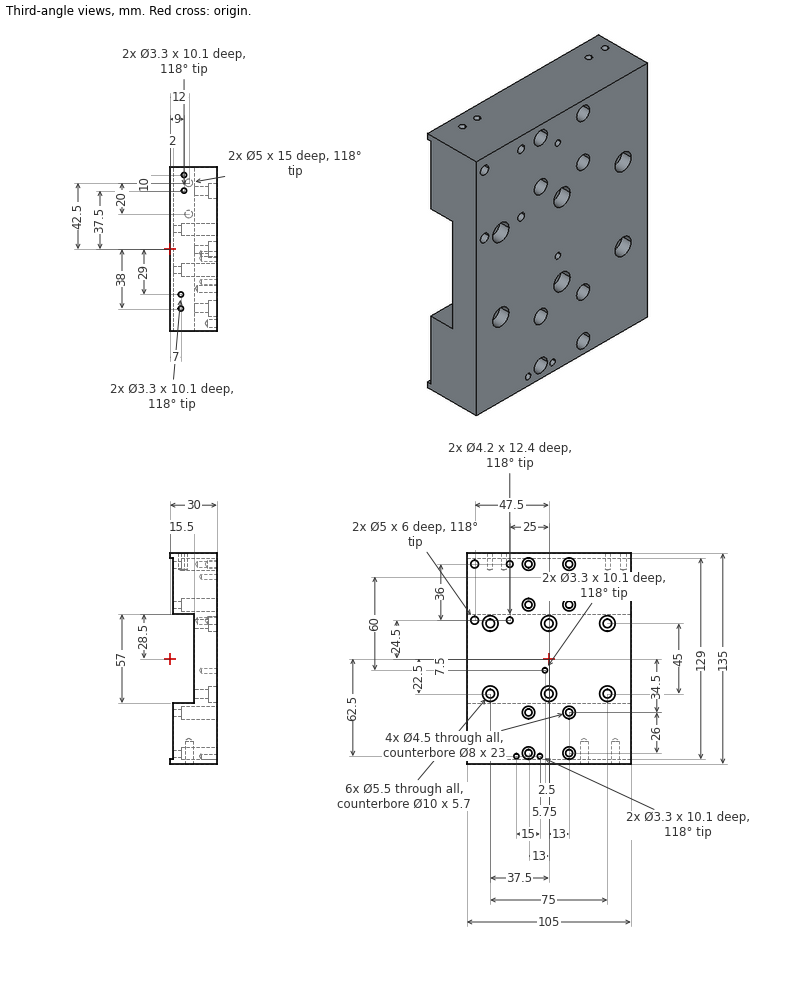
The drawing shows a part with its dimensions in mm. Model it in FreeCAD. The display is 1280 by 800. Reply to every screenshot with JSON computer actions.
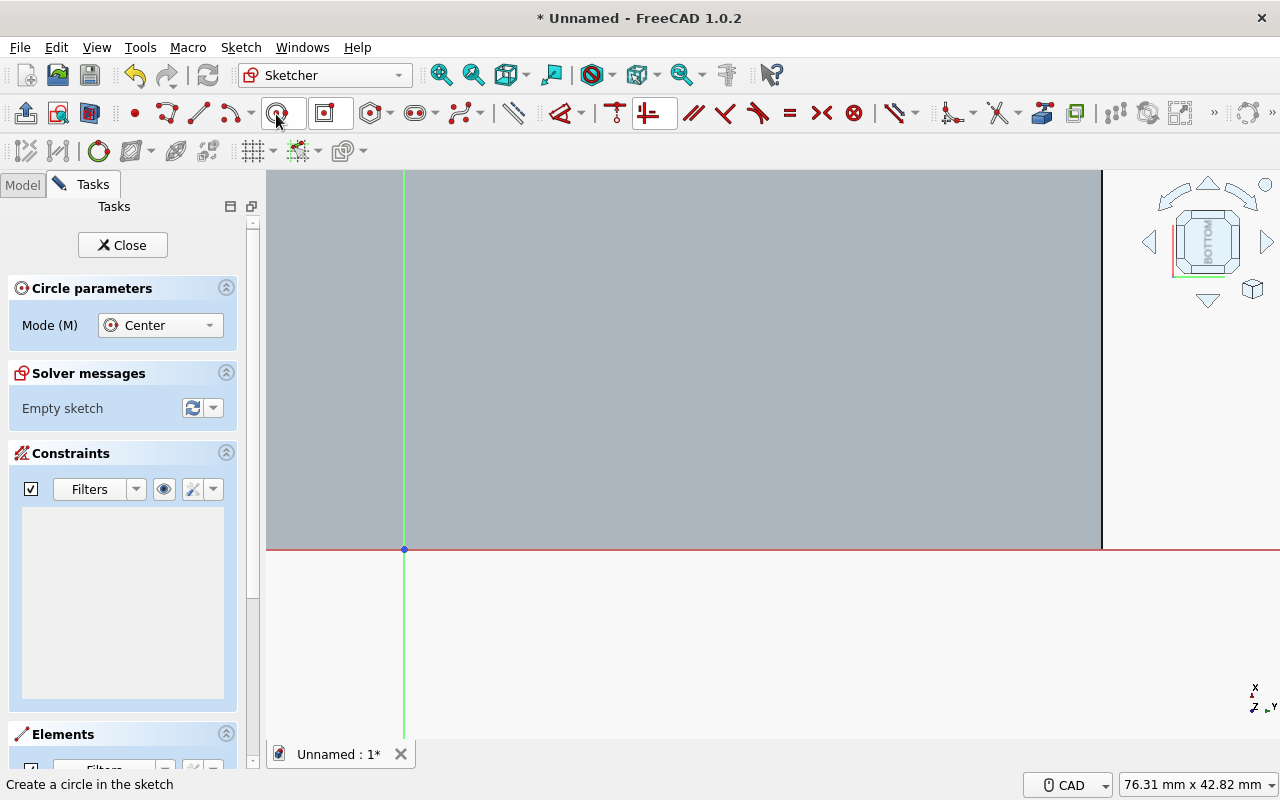
{"action": "left_click", "coordinate": [969, 390]}
{"action": "left_click", "coordinate": [993, 367]}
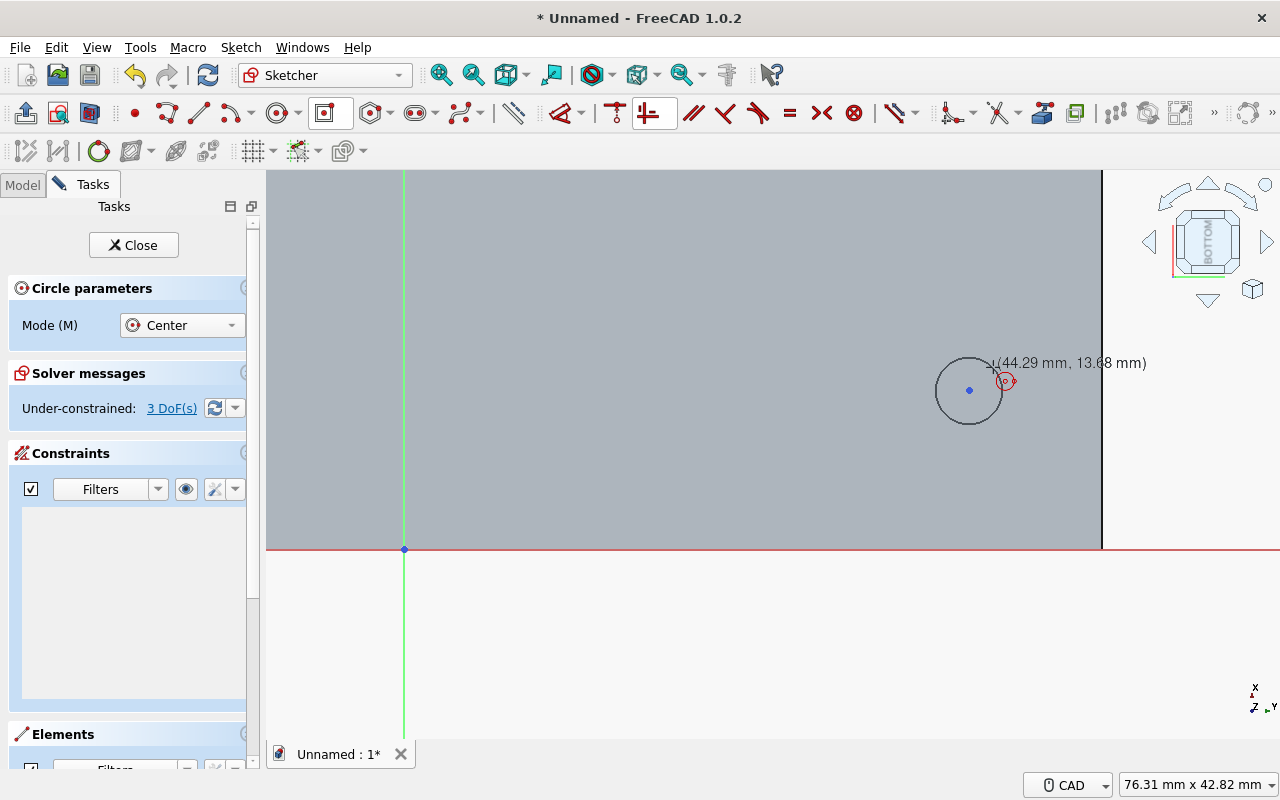
{"action": "left_click", "coordinate": [703, 390]}
{"action": "left_click", "coordinate": [727, 367]}
{"action": "key", "text": "Escape"}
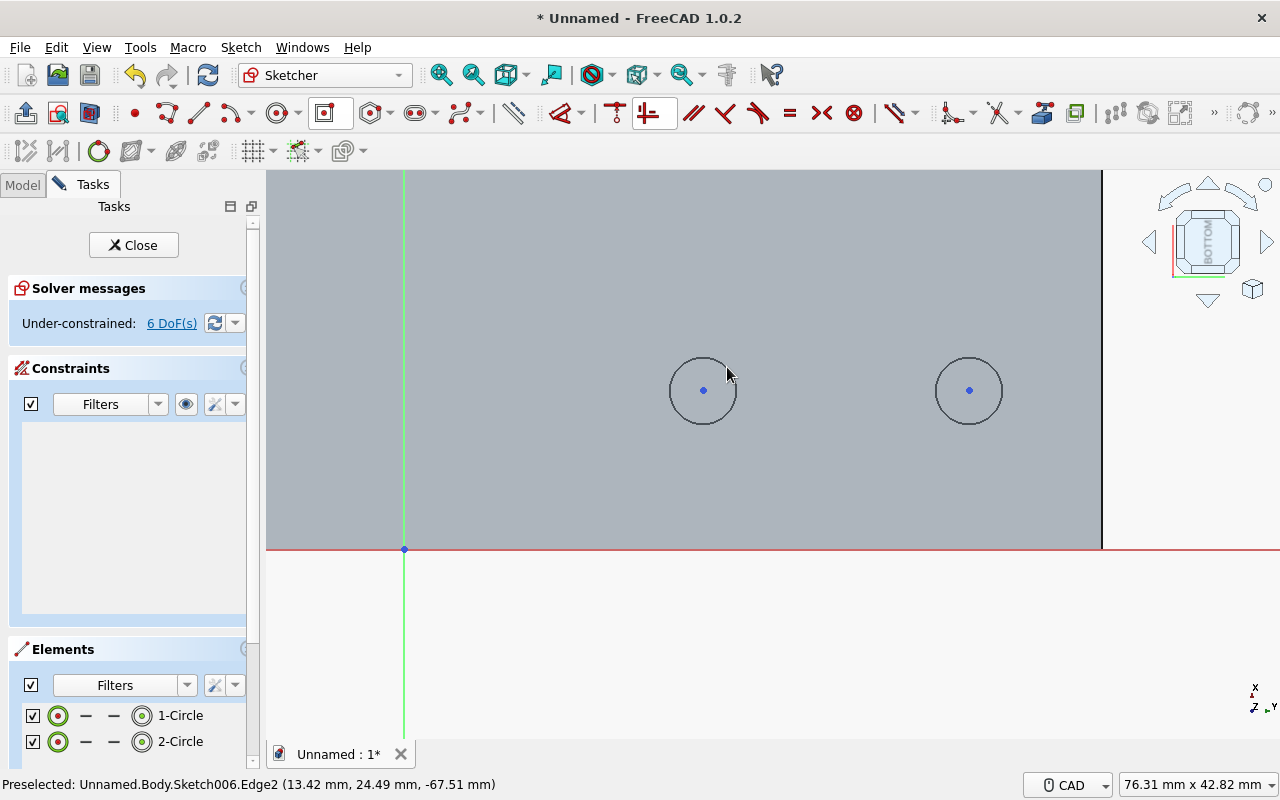
{"action": "left_click", "coordinate": [992, 367]}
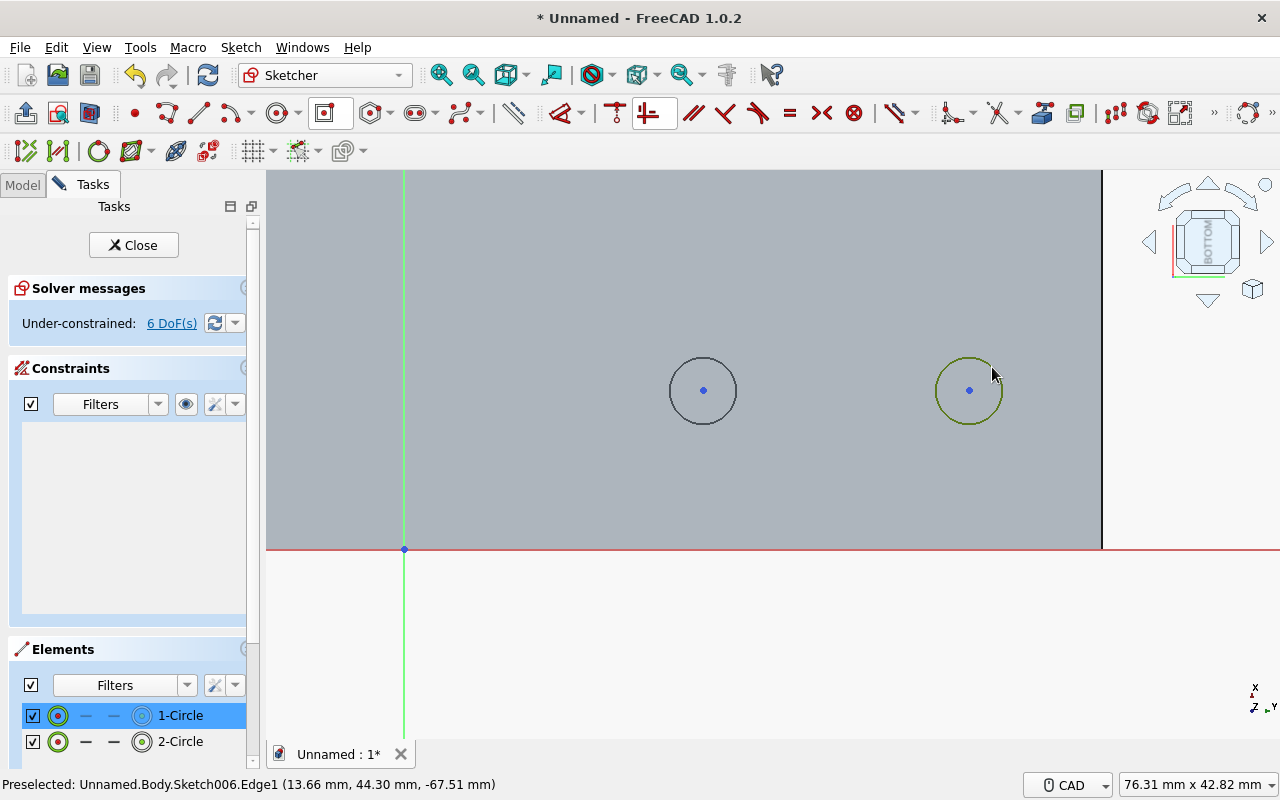
{"action": "left_click", "coordinate": [726, 367]}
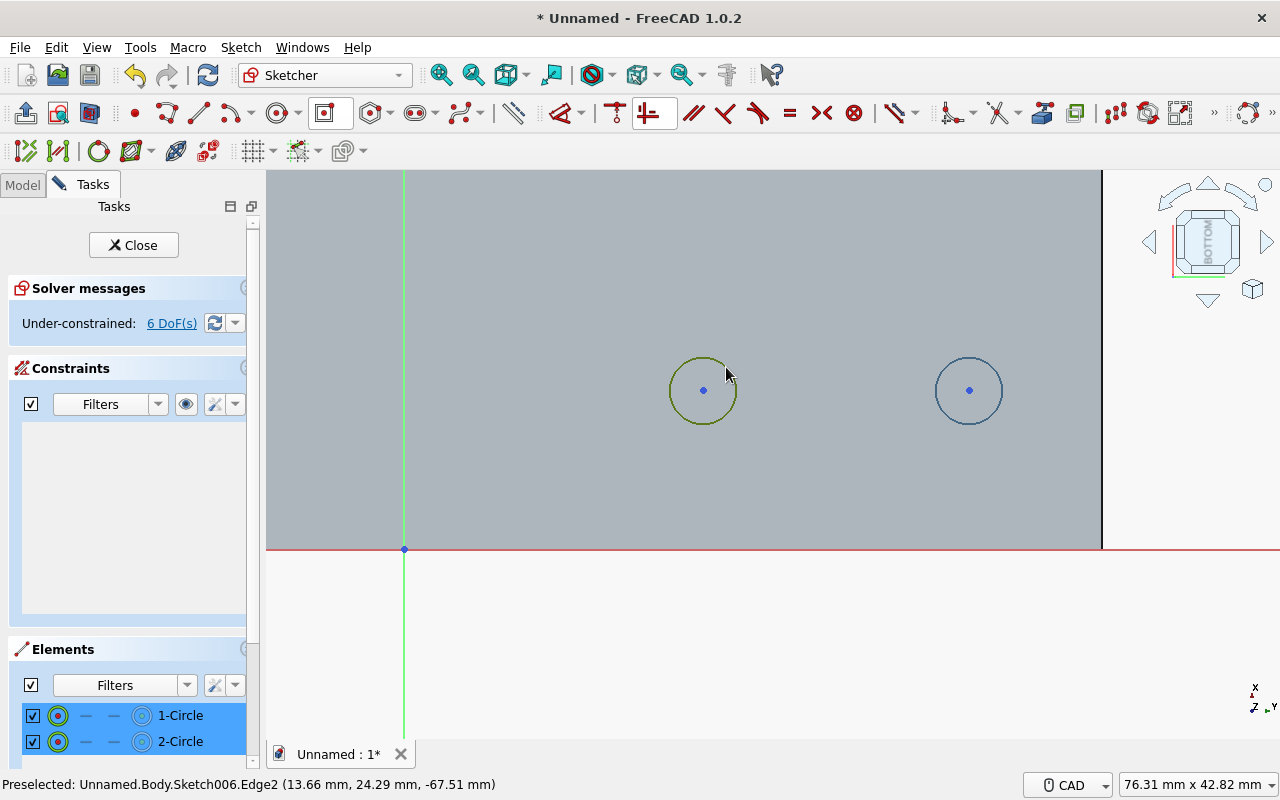
{"action": "left_click", "coordinate": [790, 114]}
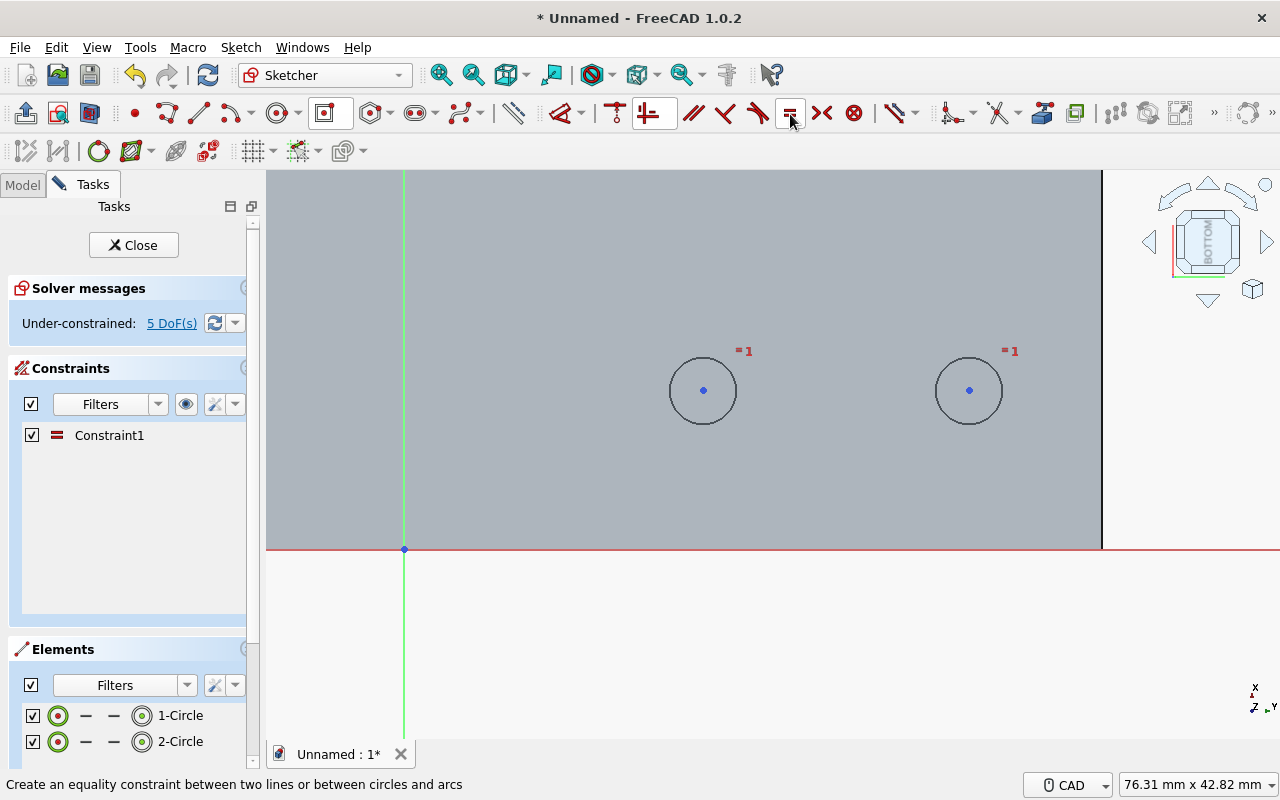
{"action": "left_click", "coordinate": [969, 391]}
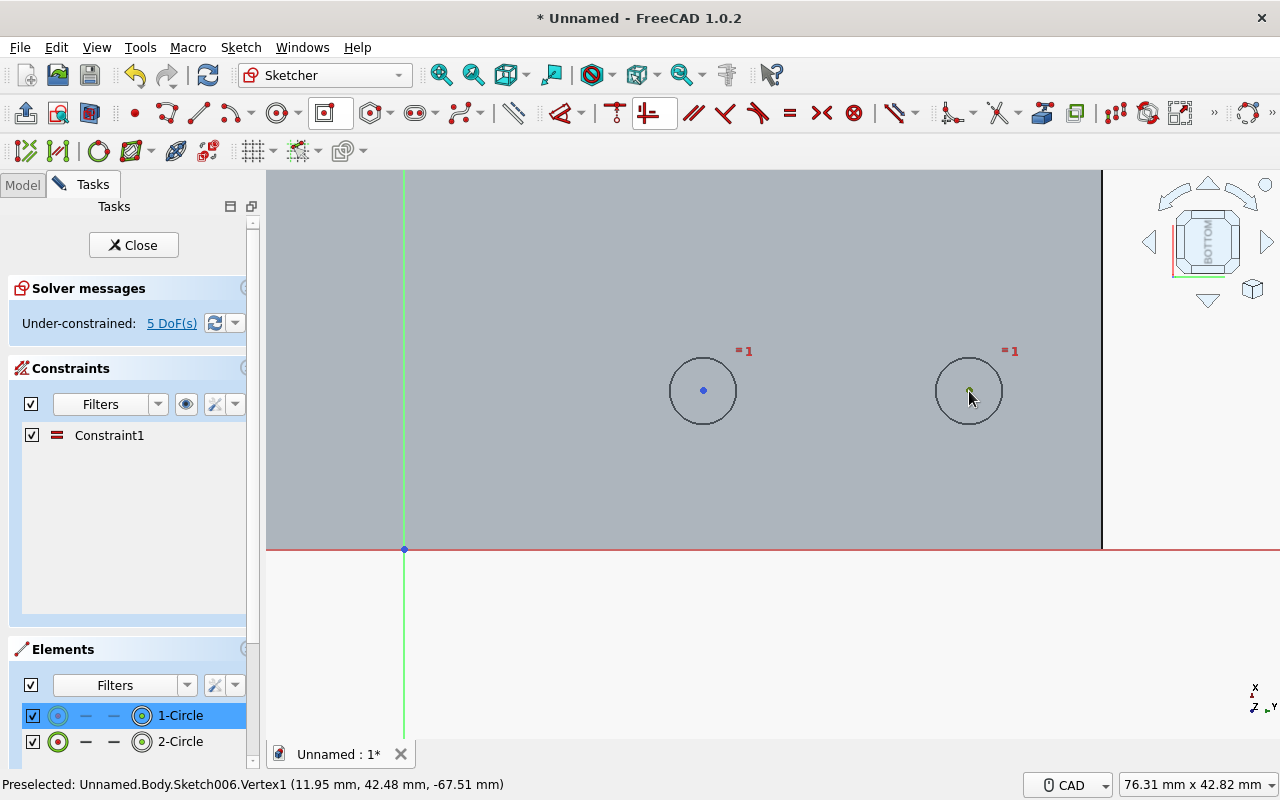
{"action": "left_click", "coordinate": [703, 391]}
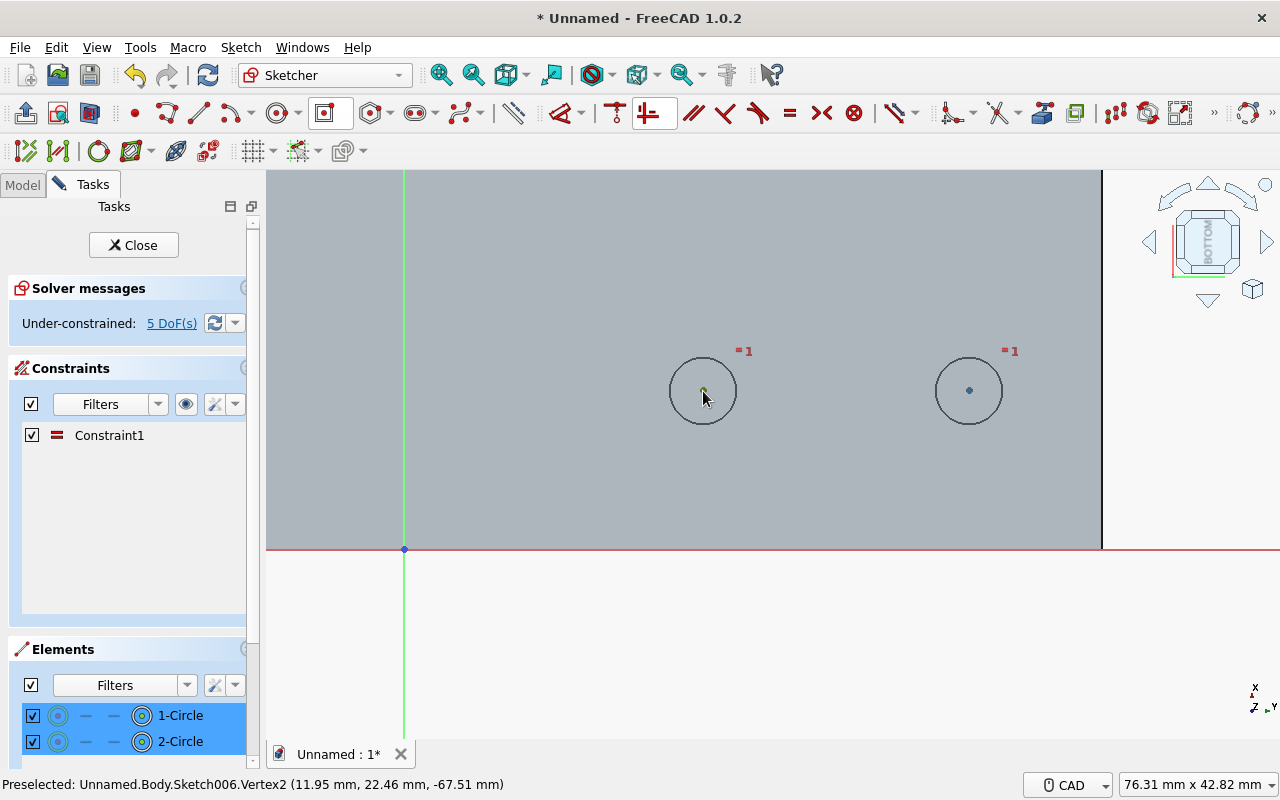
{"action": "left_click", "coordinate": [672, 114]}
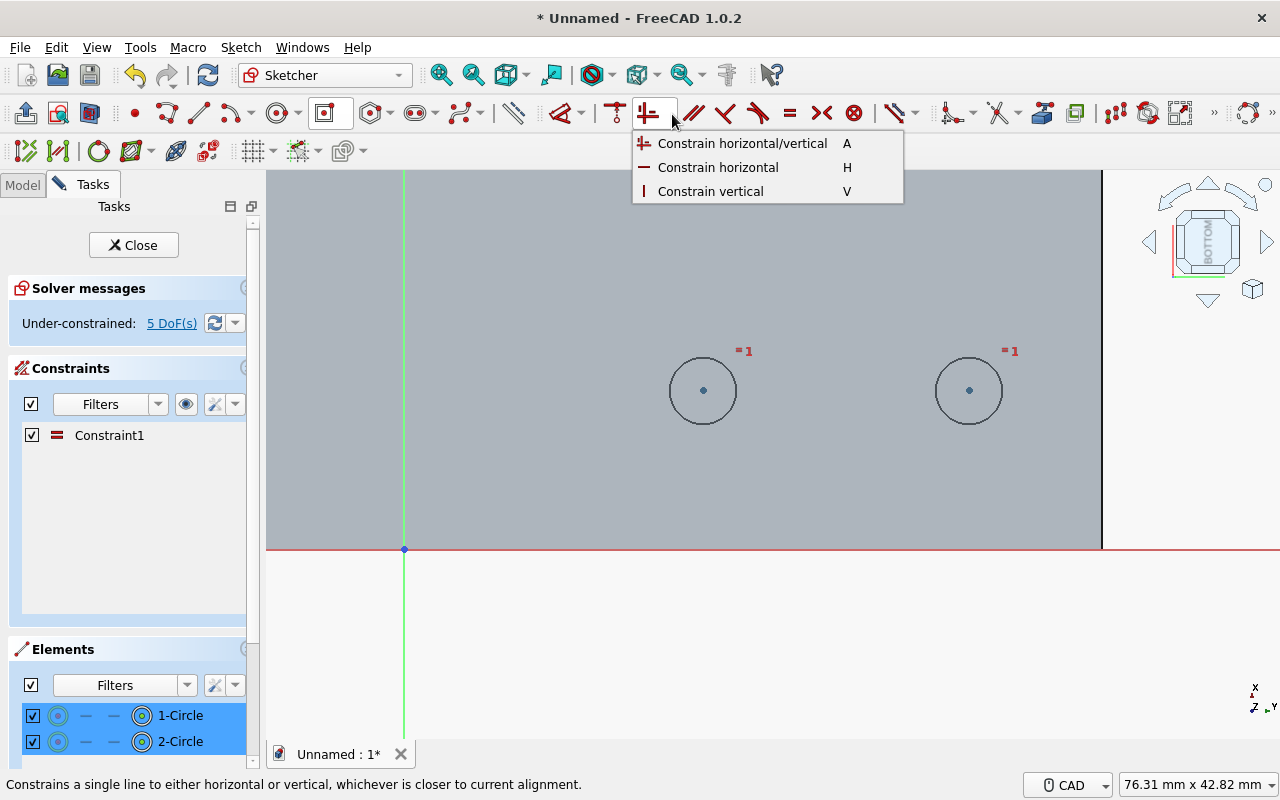
{"action": "left_click", "coordinate": [768, 167]}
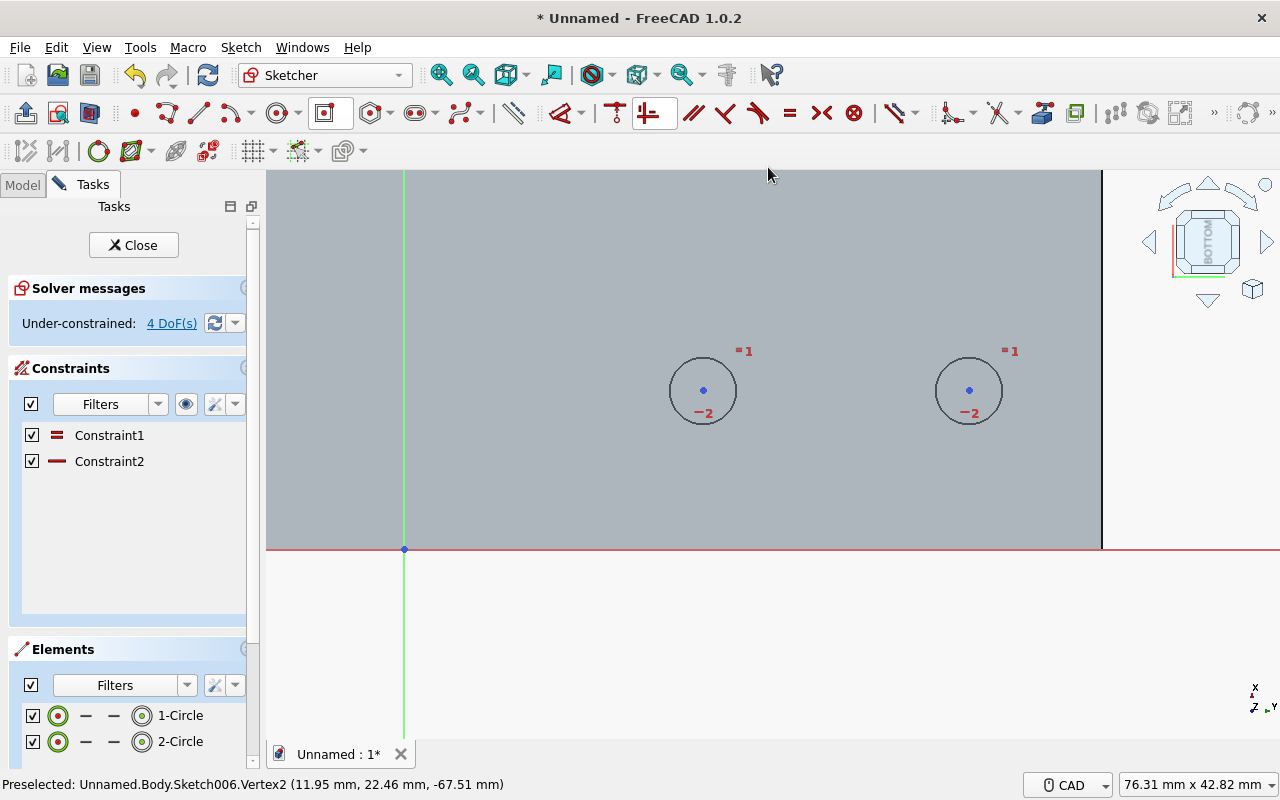
{"action": "left_click", "coordinate": [560, 114]}